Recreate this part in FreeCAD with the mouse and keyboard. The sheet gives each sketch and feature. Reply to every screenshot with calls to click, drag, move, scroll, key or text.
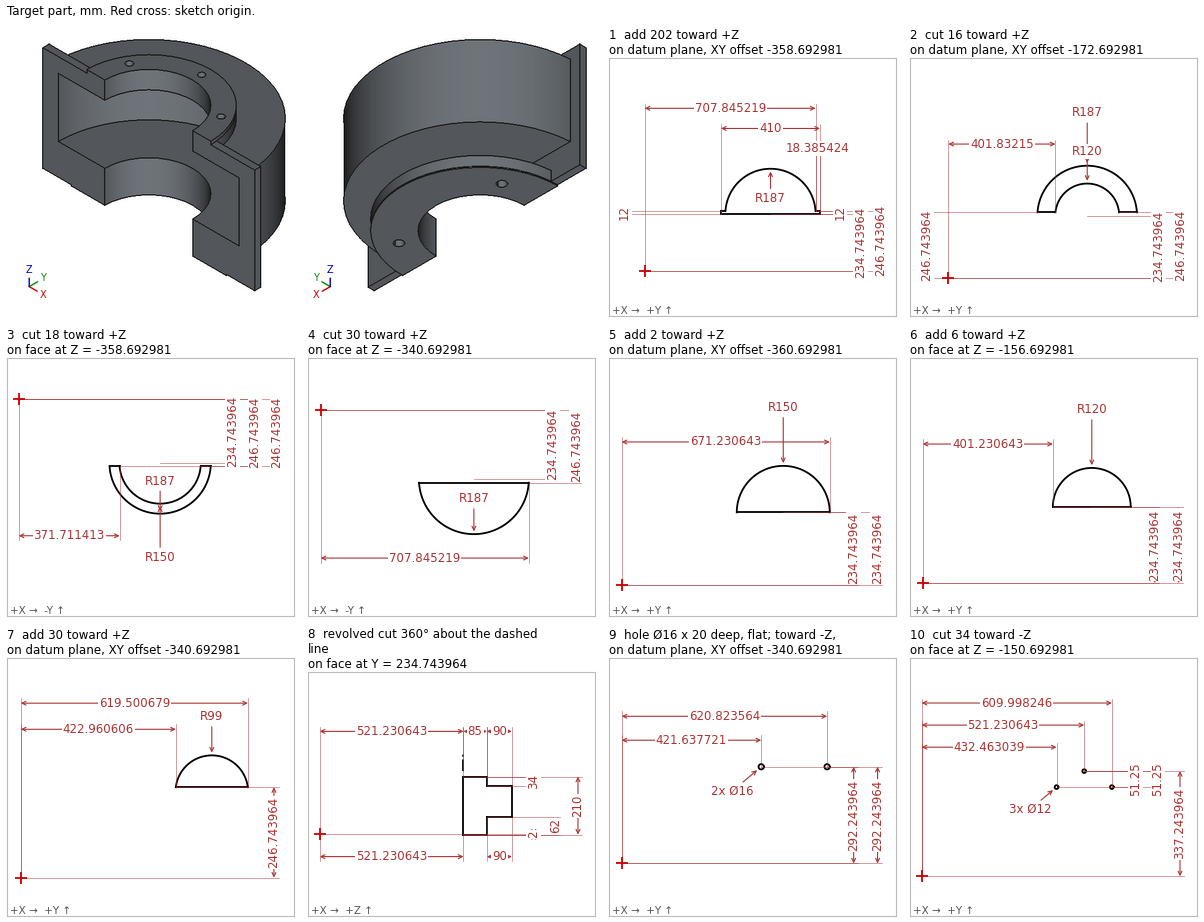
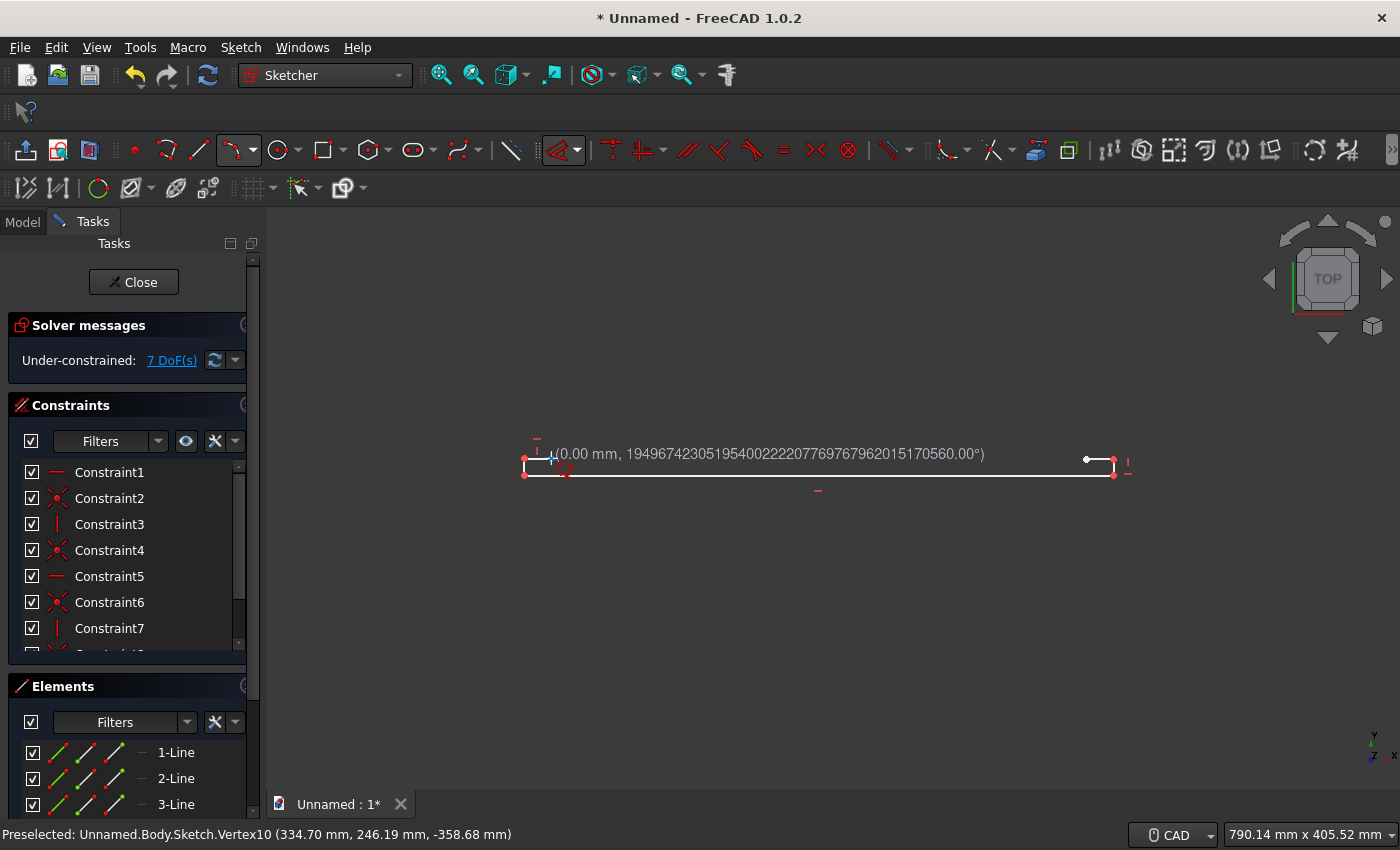
click(232, 150)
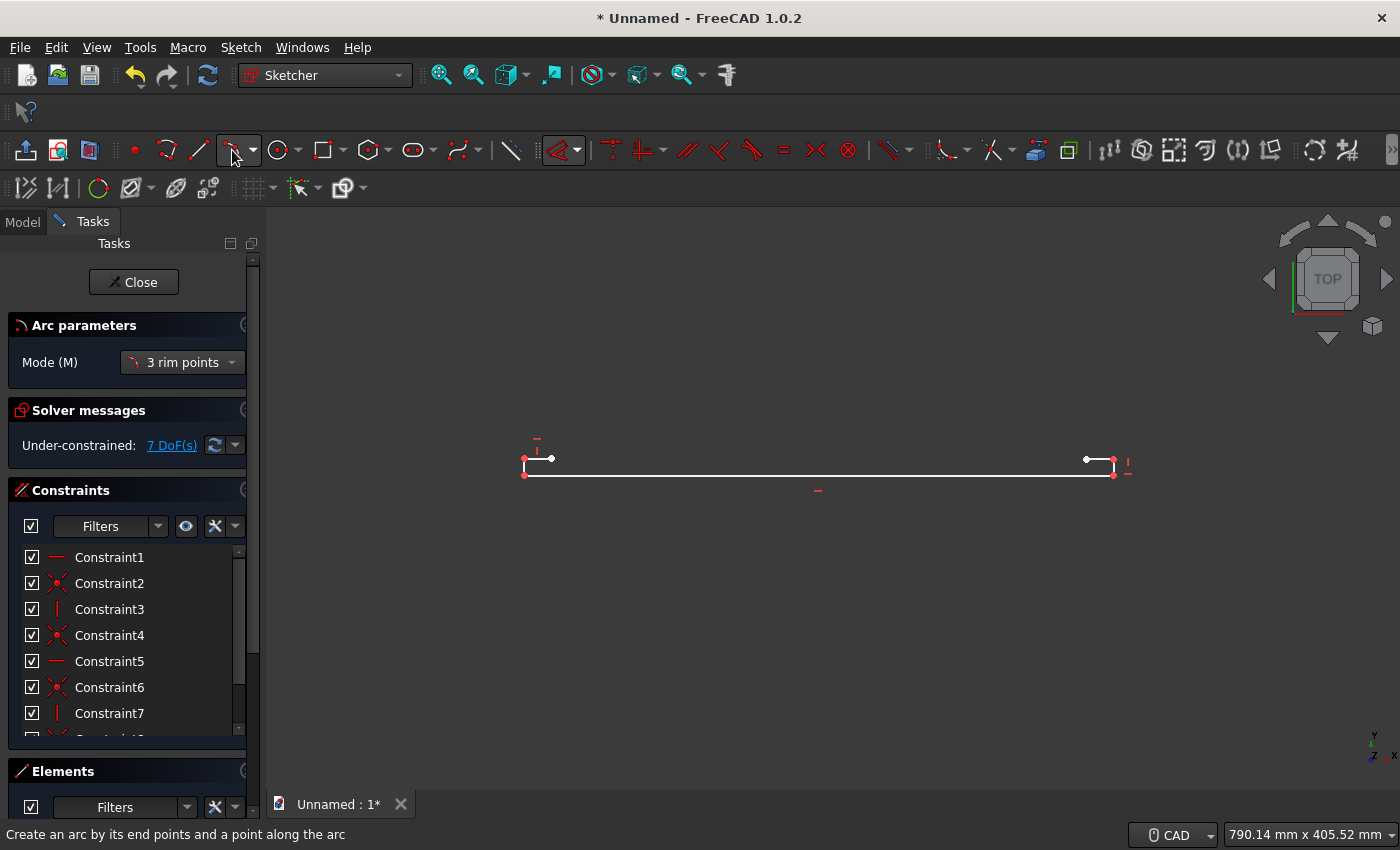
click(551, 459)
click(1087, 459)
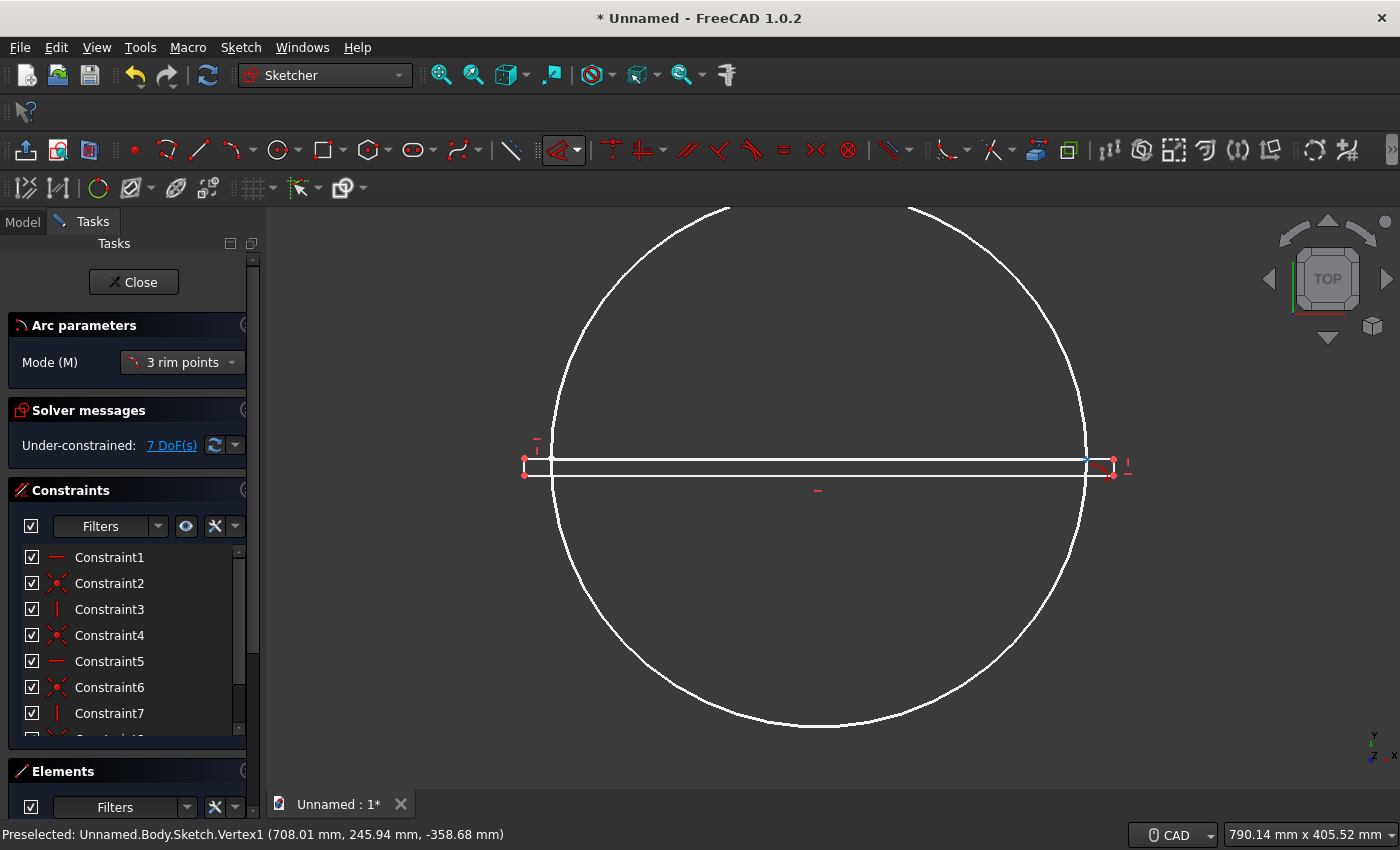
scroll(1116, 474, down, 2)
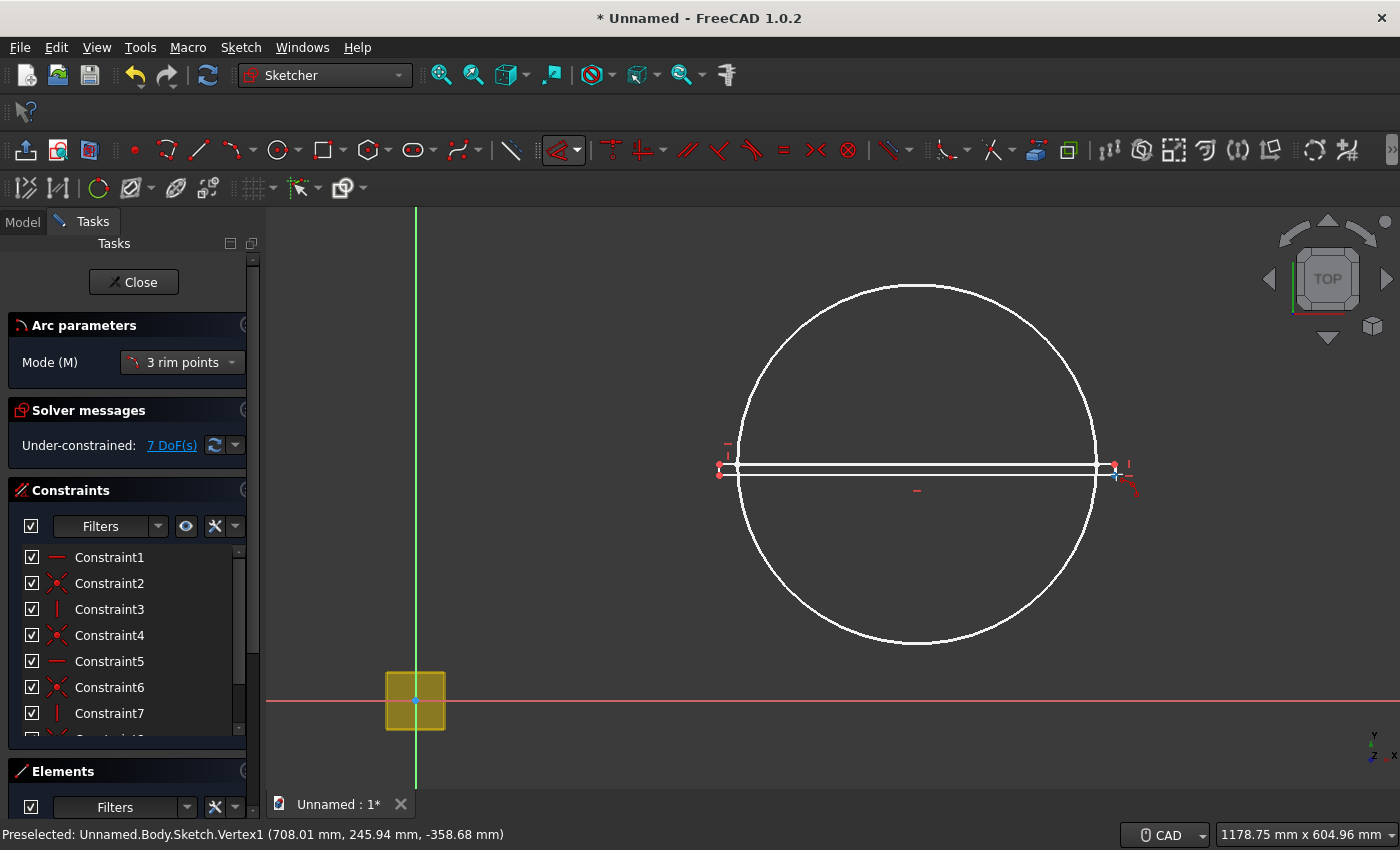
click(917, 295)
key(Escape)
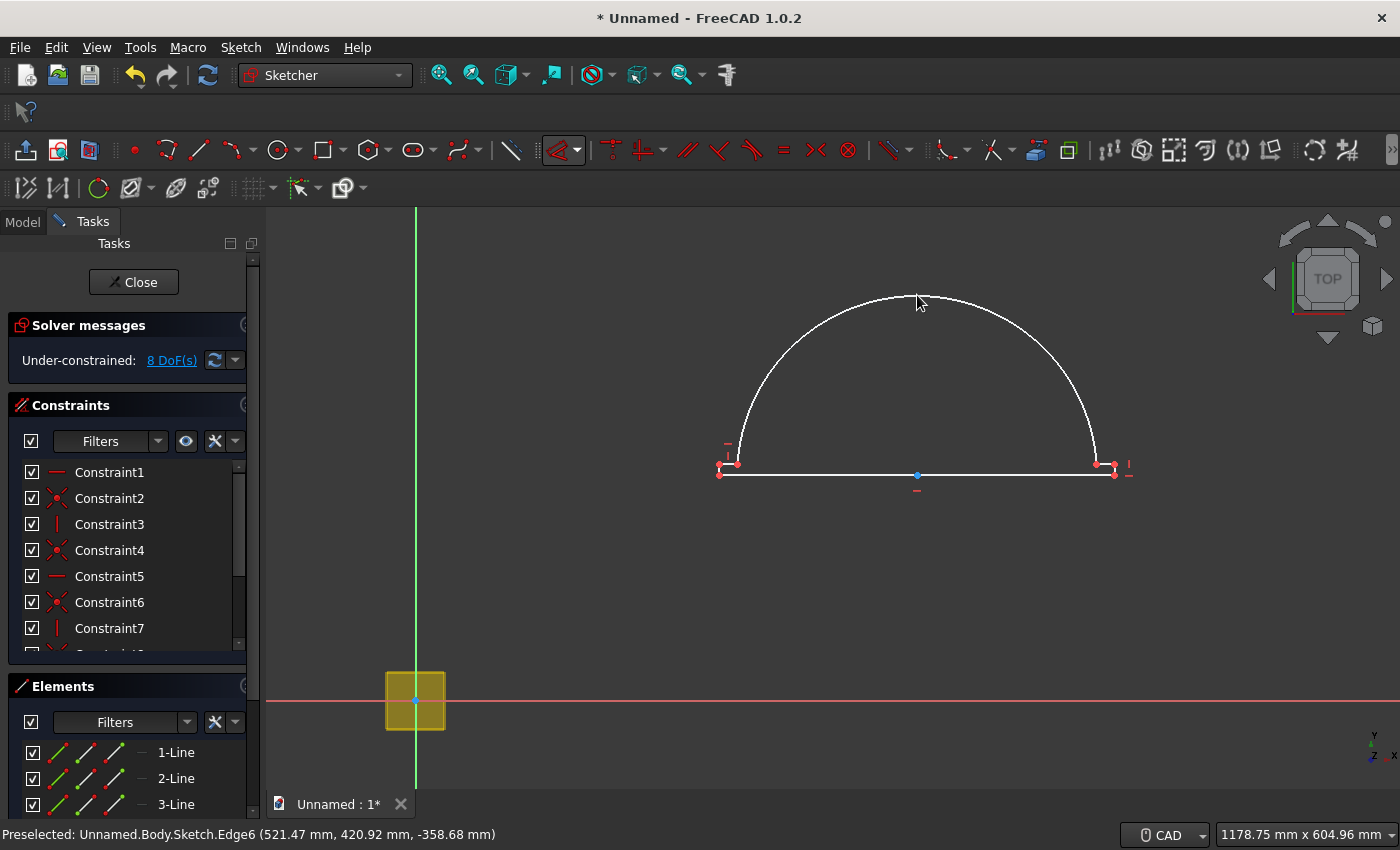
key(d)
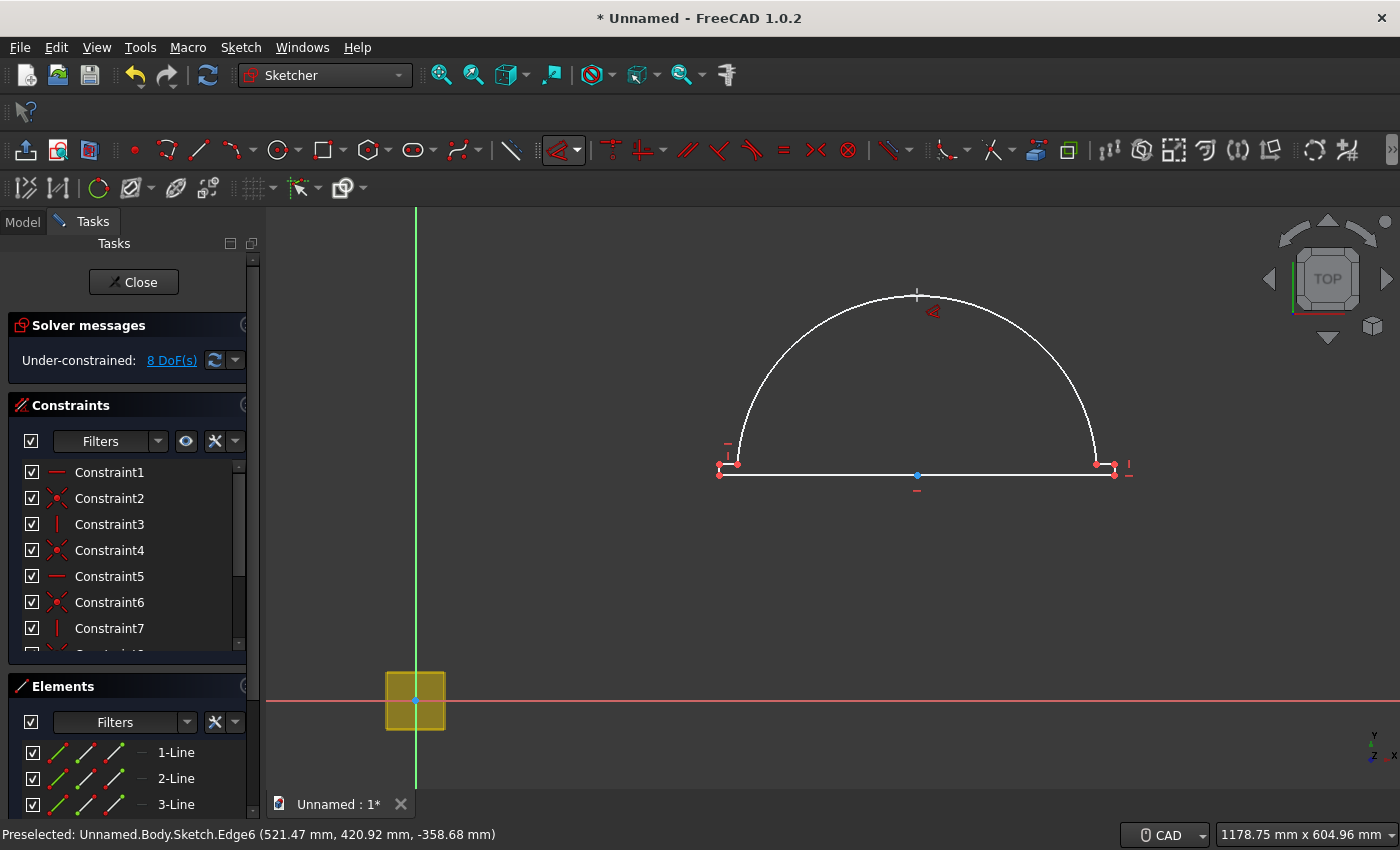
click(1019, 328)
click(1037, 302)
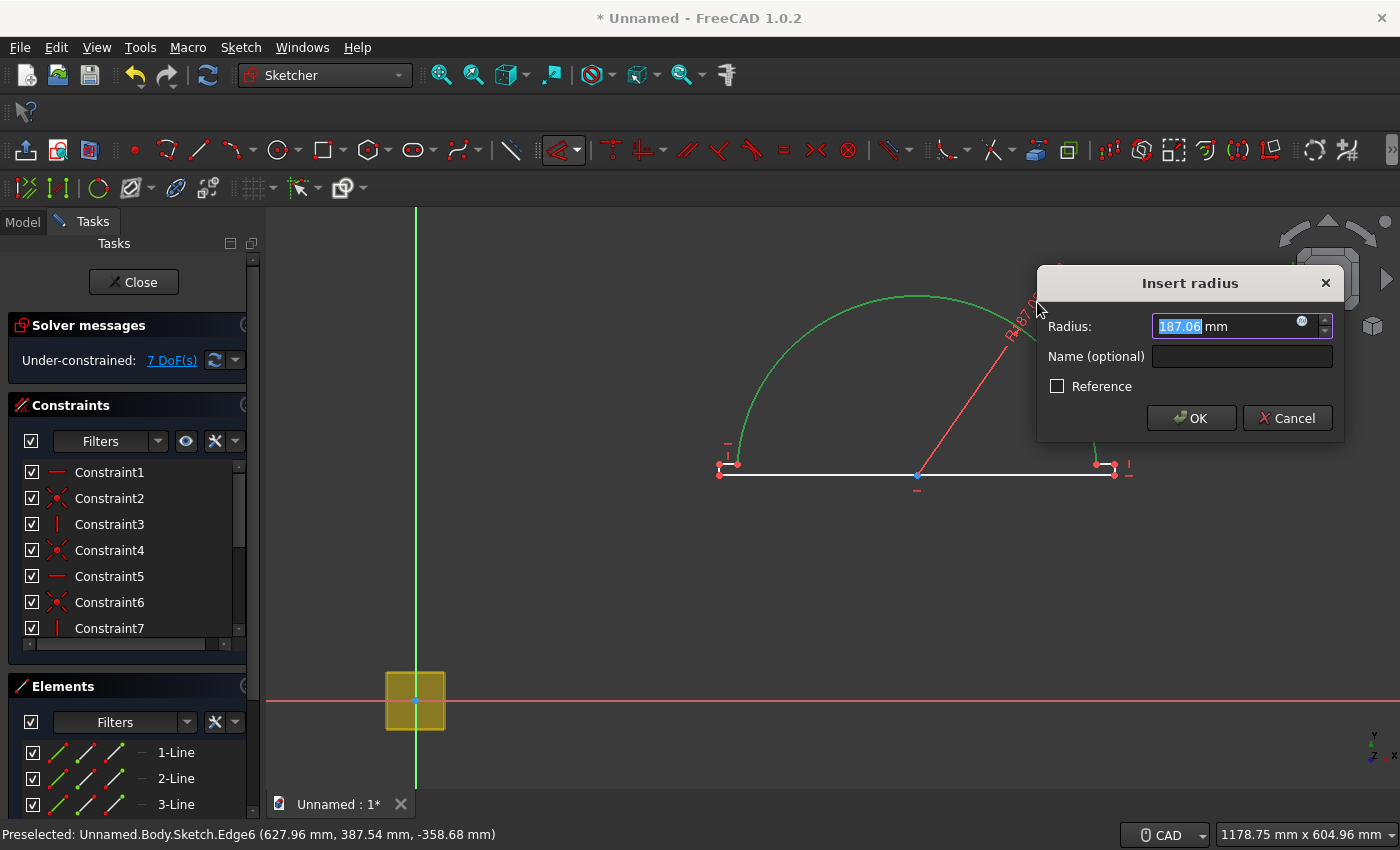
text(187)
key(Return)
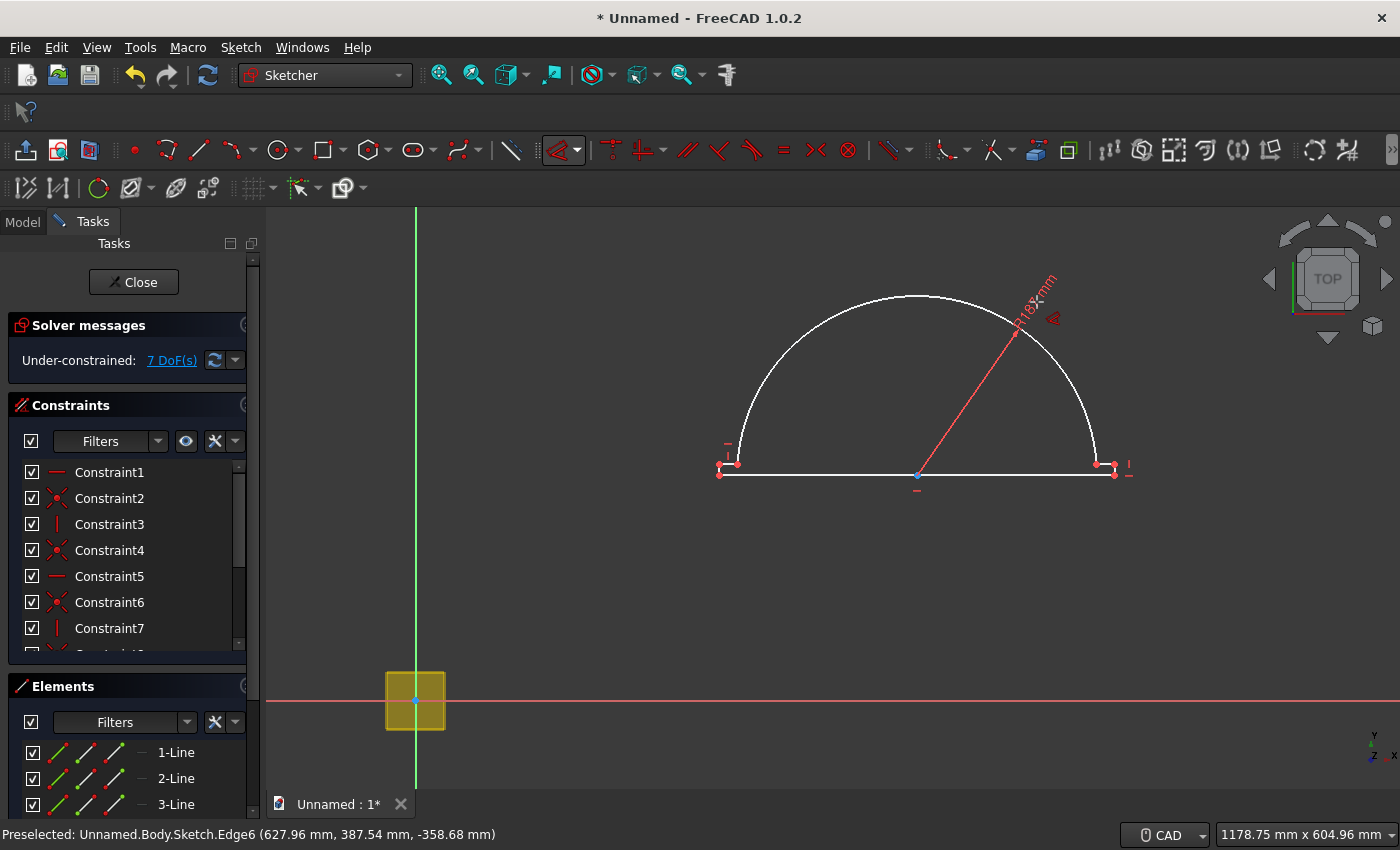
scroll(1115, 470, up, 7)